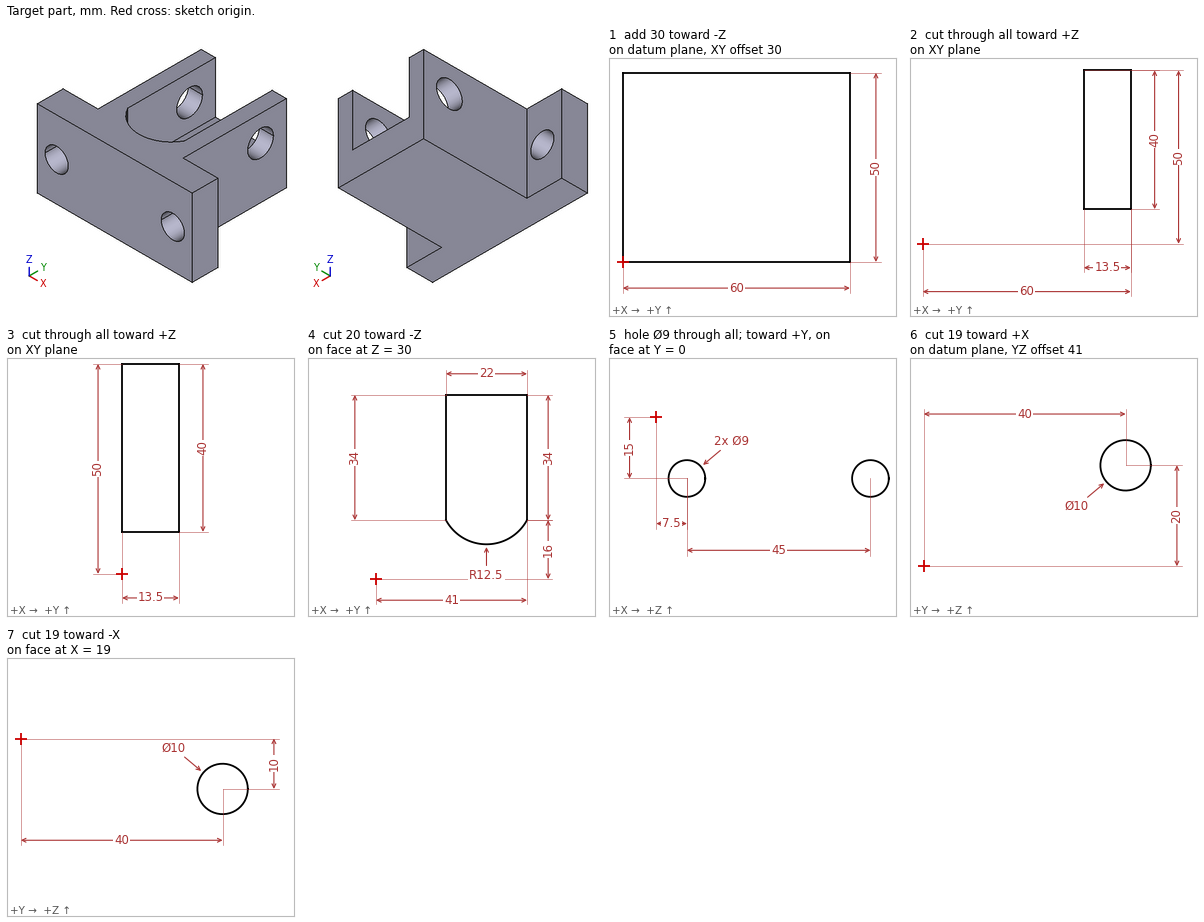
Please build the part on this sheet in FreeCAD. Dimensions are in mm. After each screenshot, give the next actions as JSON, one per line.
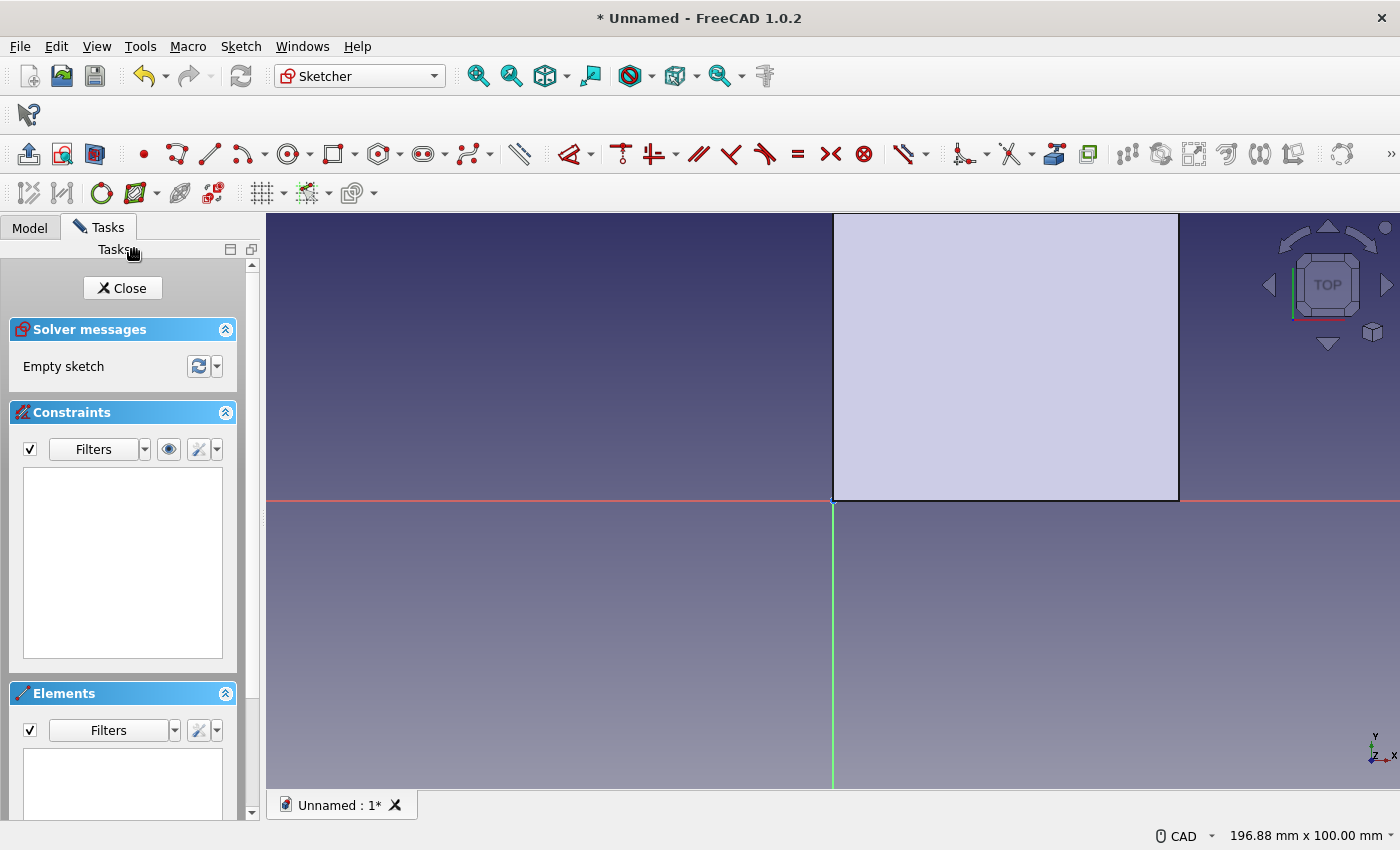
{"action": "left_click", "coordinate": [95, 154]}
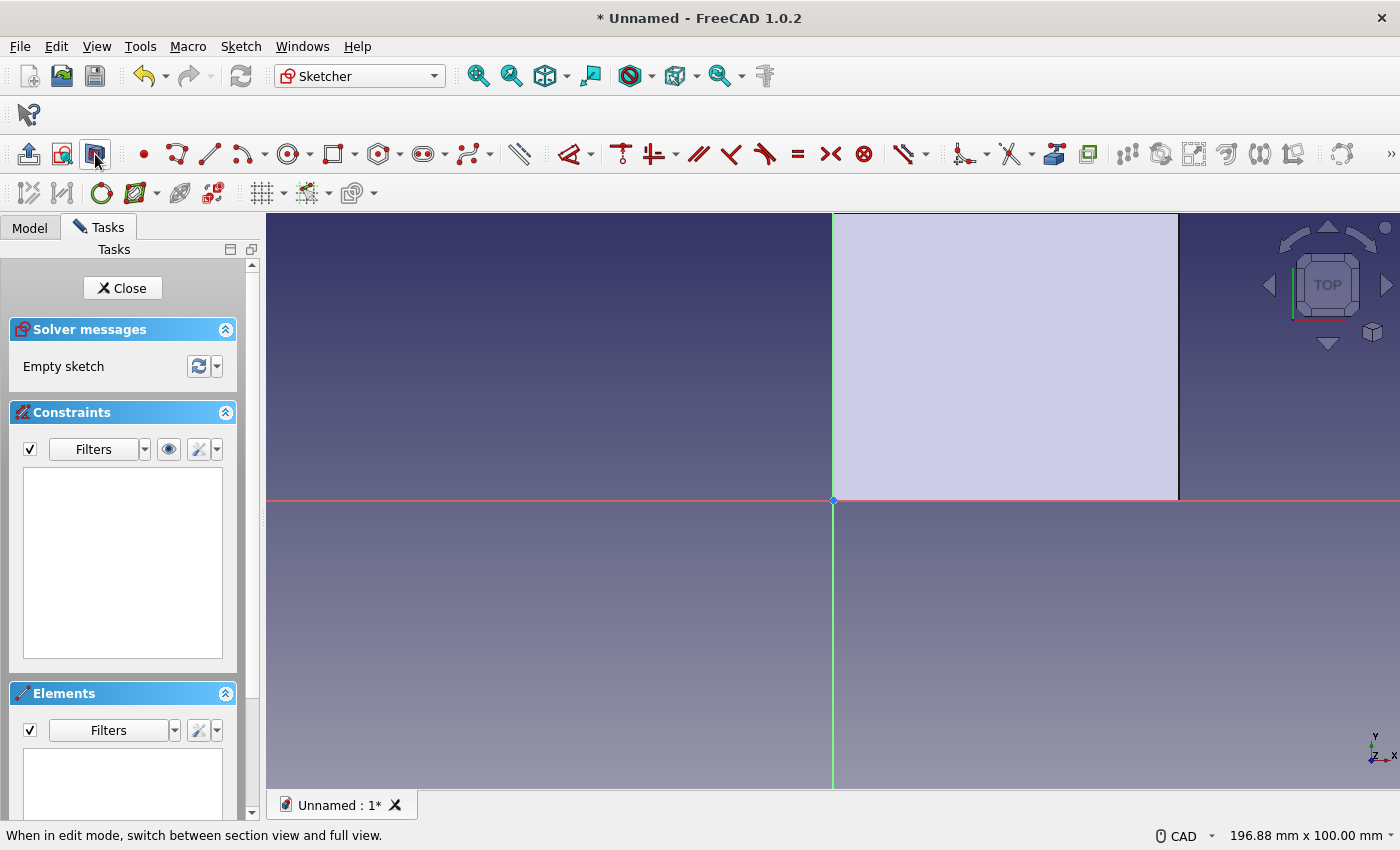
{"action": "scroll", "coordinate": [294, 761], "scroll_direction": "down", "scroll_amount": 1}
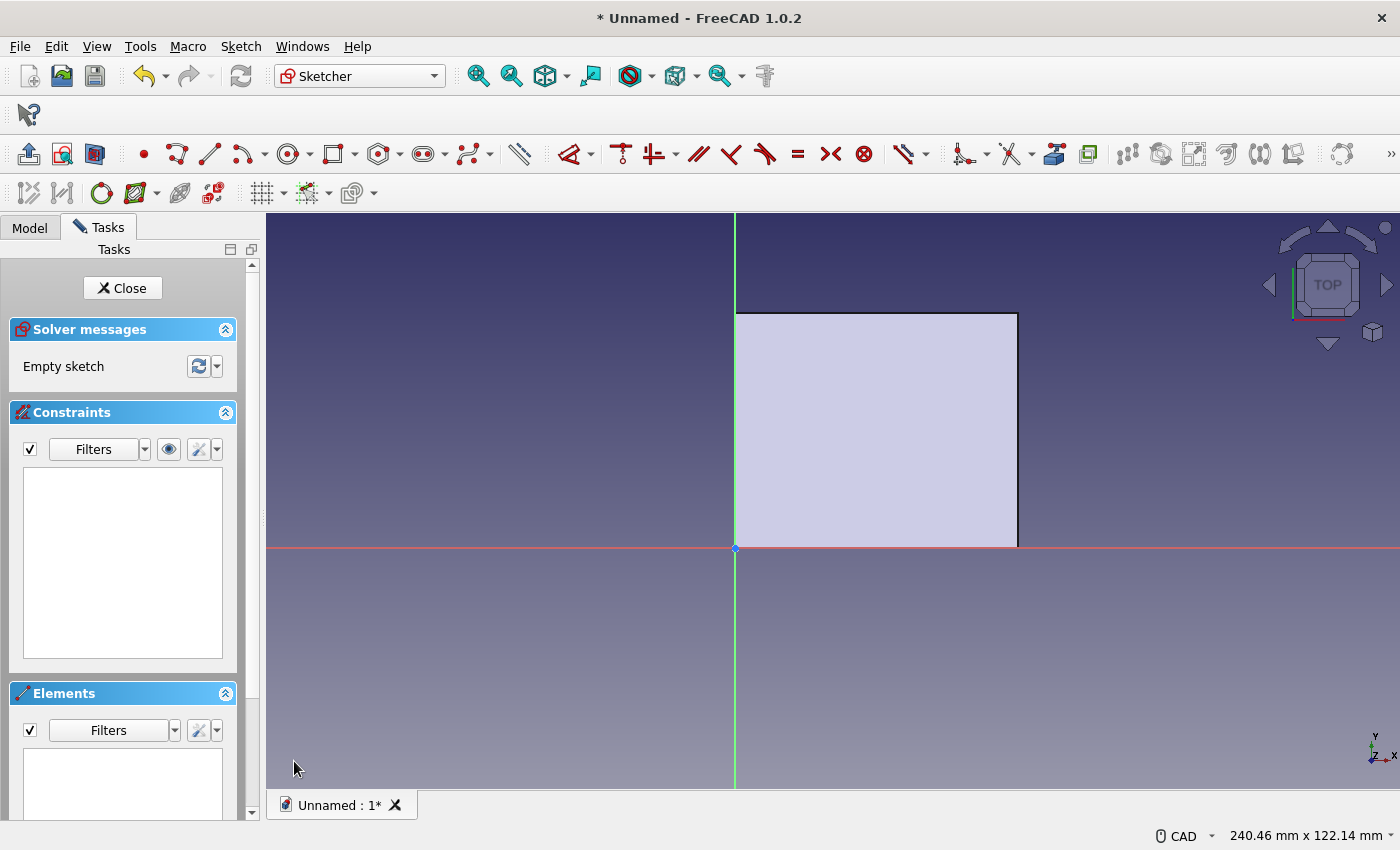
{"action": "scroll", "coordinate": [1105, 287], "scroll_direction": "up", "scroll_amount": 2}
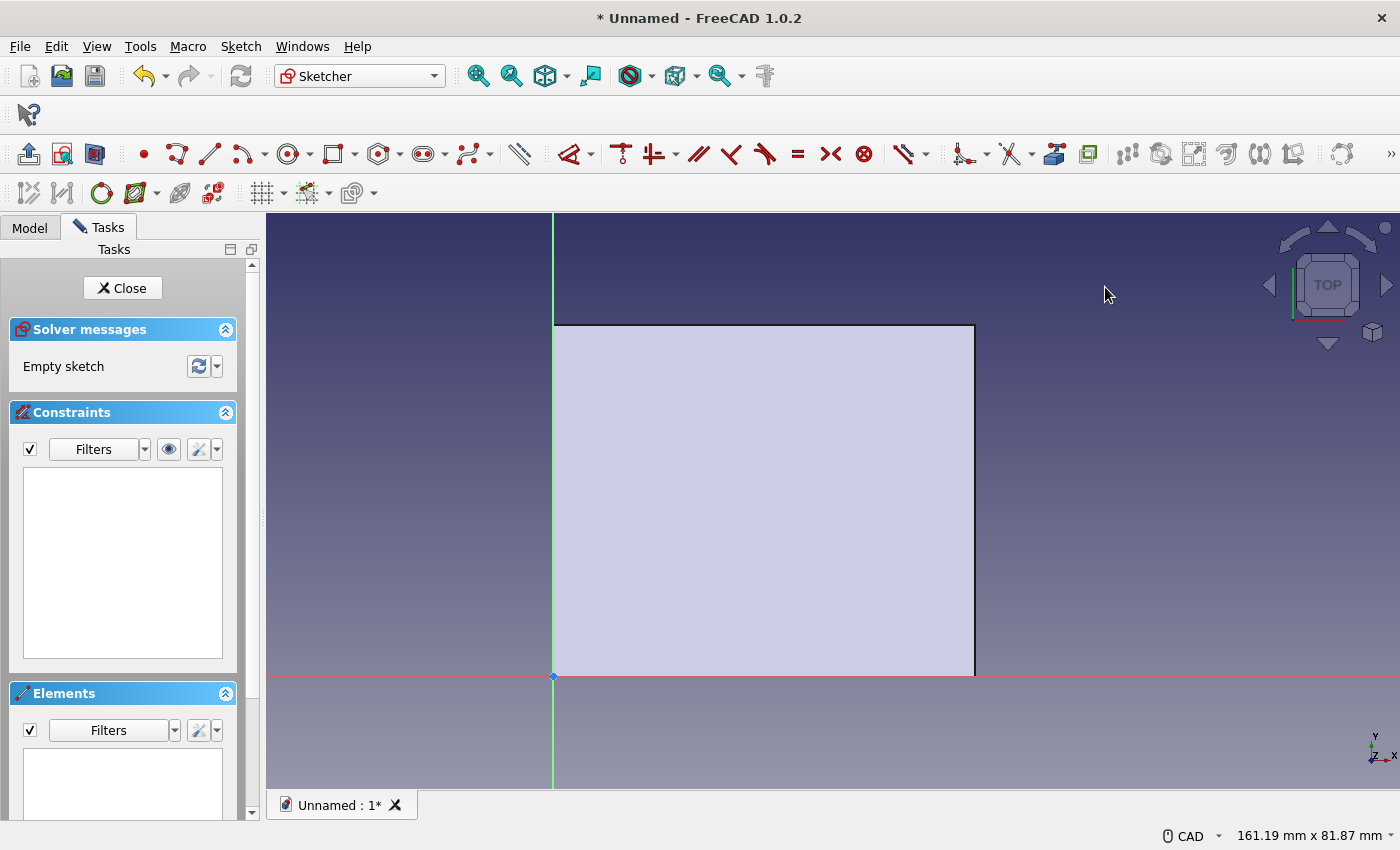
{"action": "key", "text": "g r"}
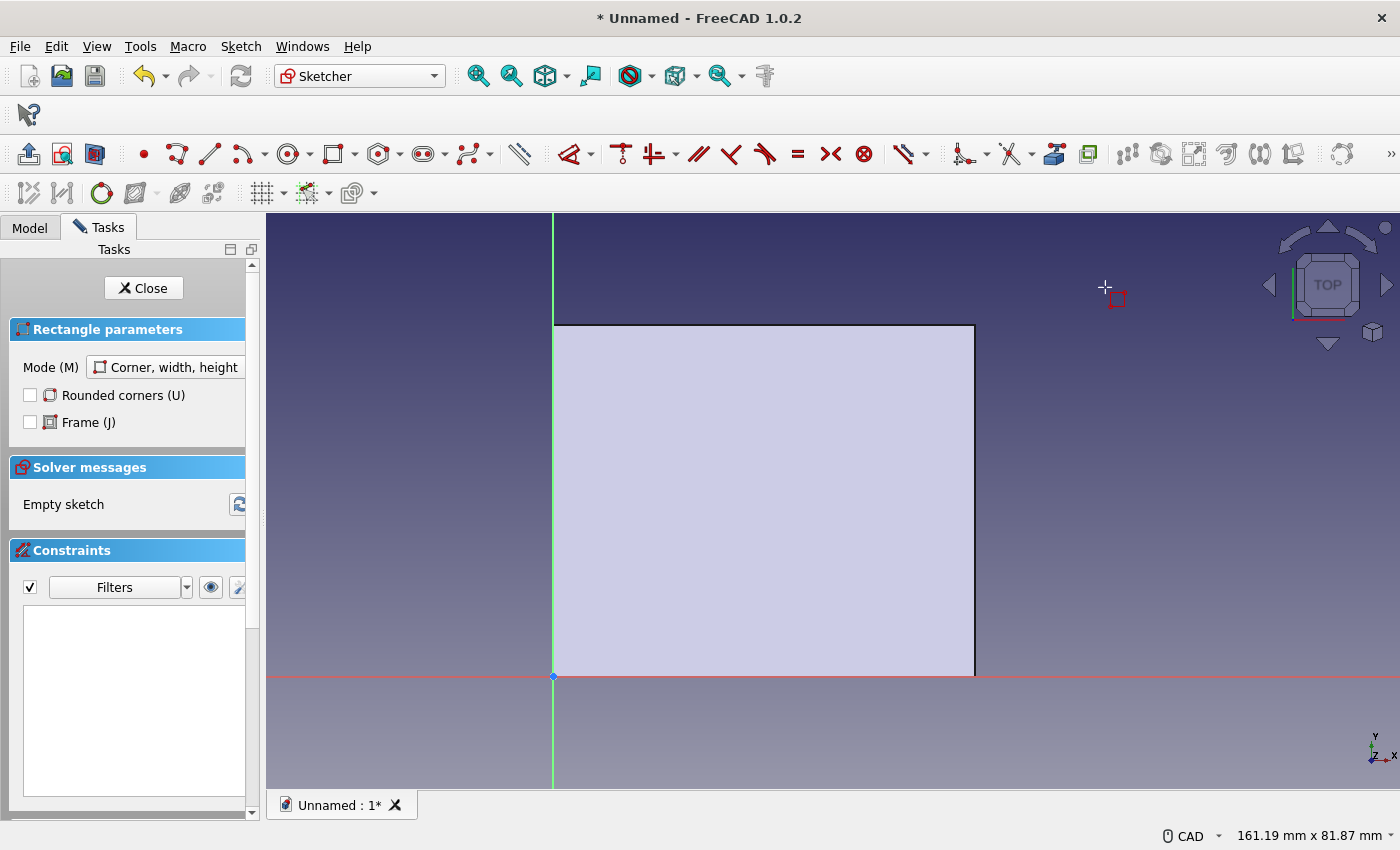
{"action": "left_click", "coordinate": [880, 325]}
{"action": "mouse_move", "coordinate": [975, 606]}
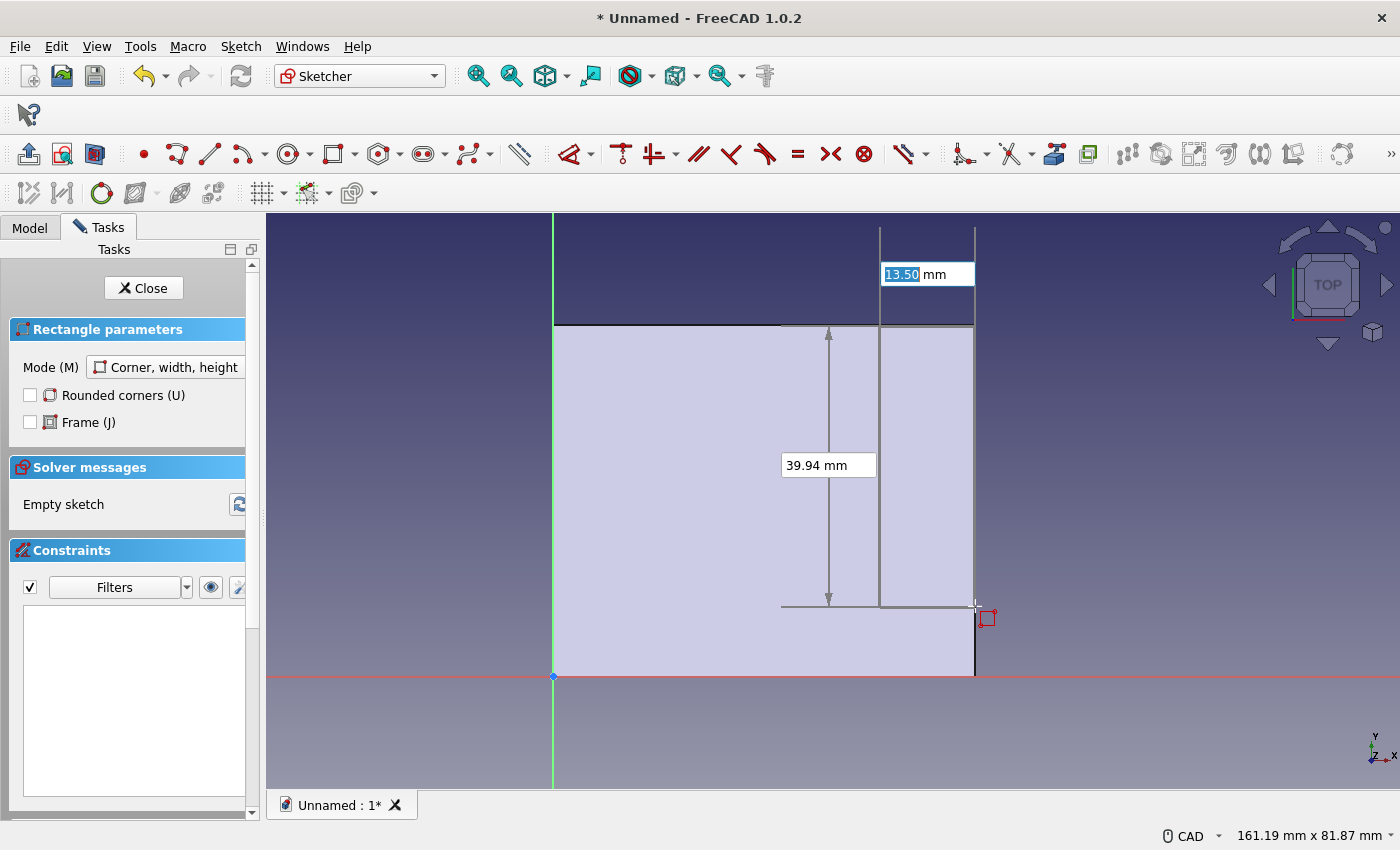
{"action": "type", "text": "13.5"}
{"action": "key", "text": "Tab"}
{"action": "type", "text": "40"}
{"action": "key", "text": "Return"}
{"action": "key", "text": "Escape"}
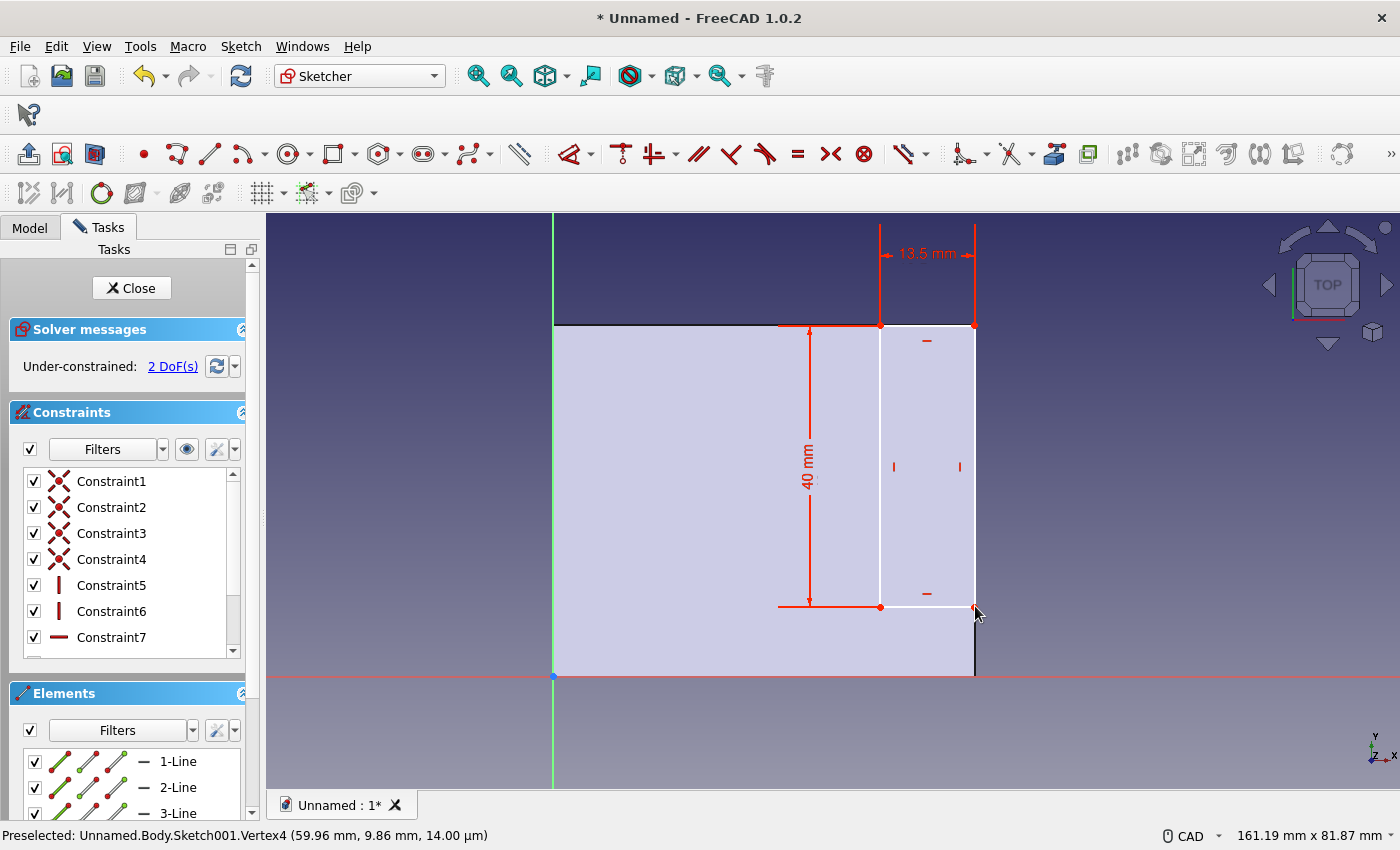
{"action": "left_click", "coordinate": [880, 326]}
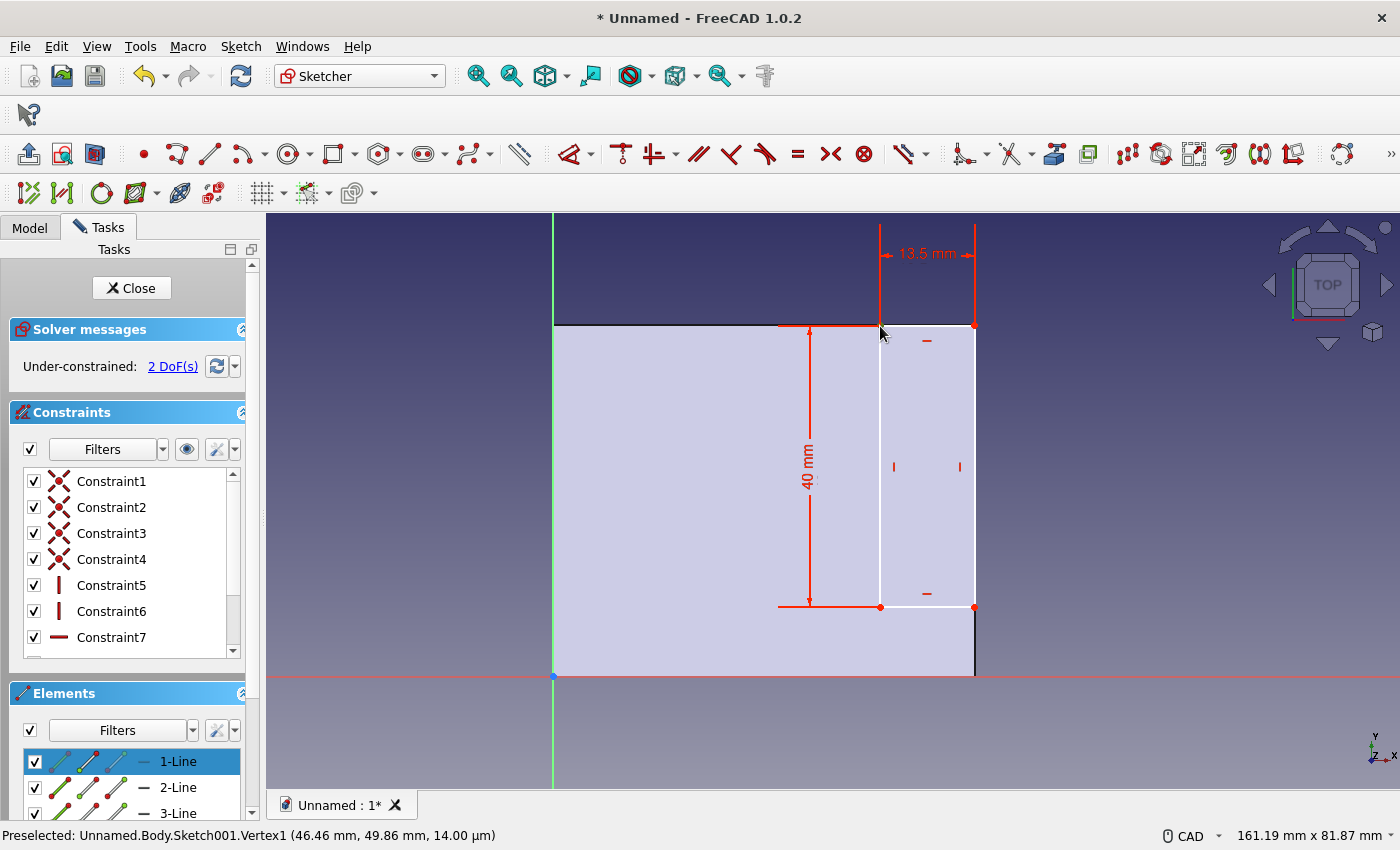
{"action": "key", "text": "i"}